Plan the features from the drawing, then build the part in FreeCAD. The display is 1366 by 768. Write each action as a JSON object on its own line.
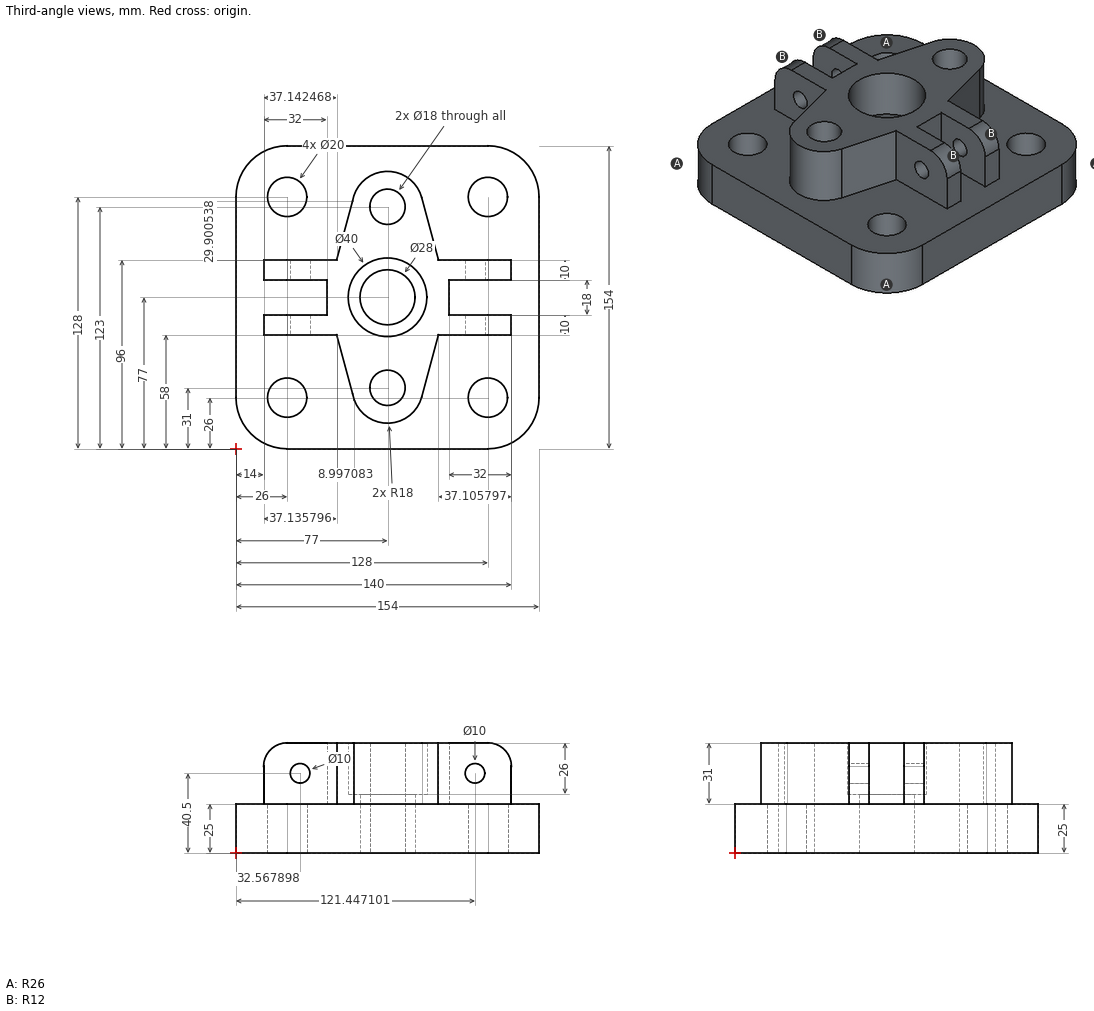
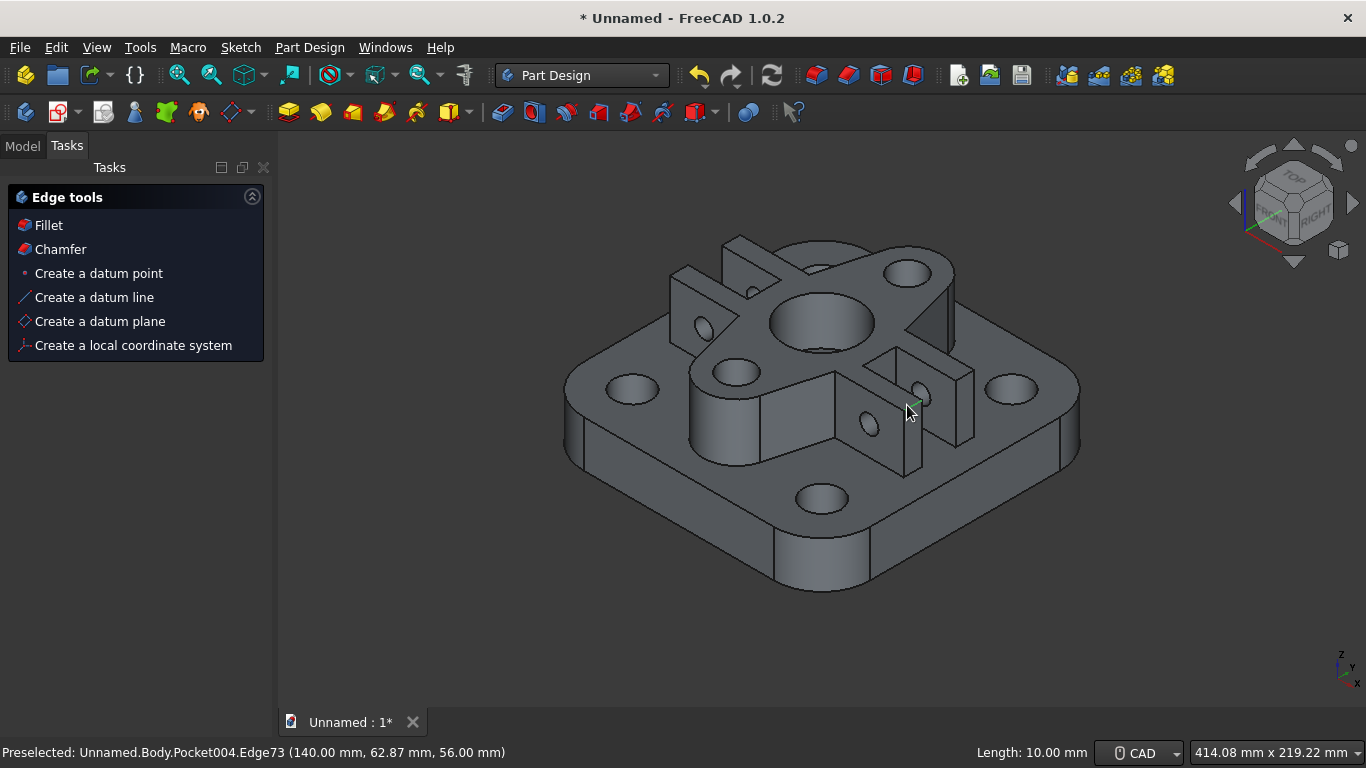
{"action": "left_click", "coordinate": [965, 374], "text": "ctrl"}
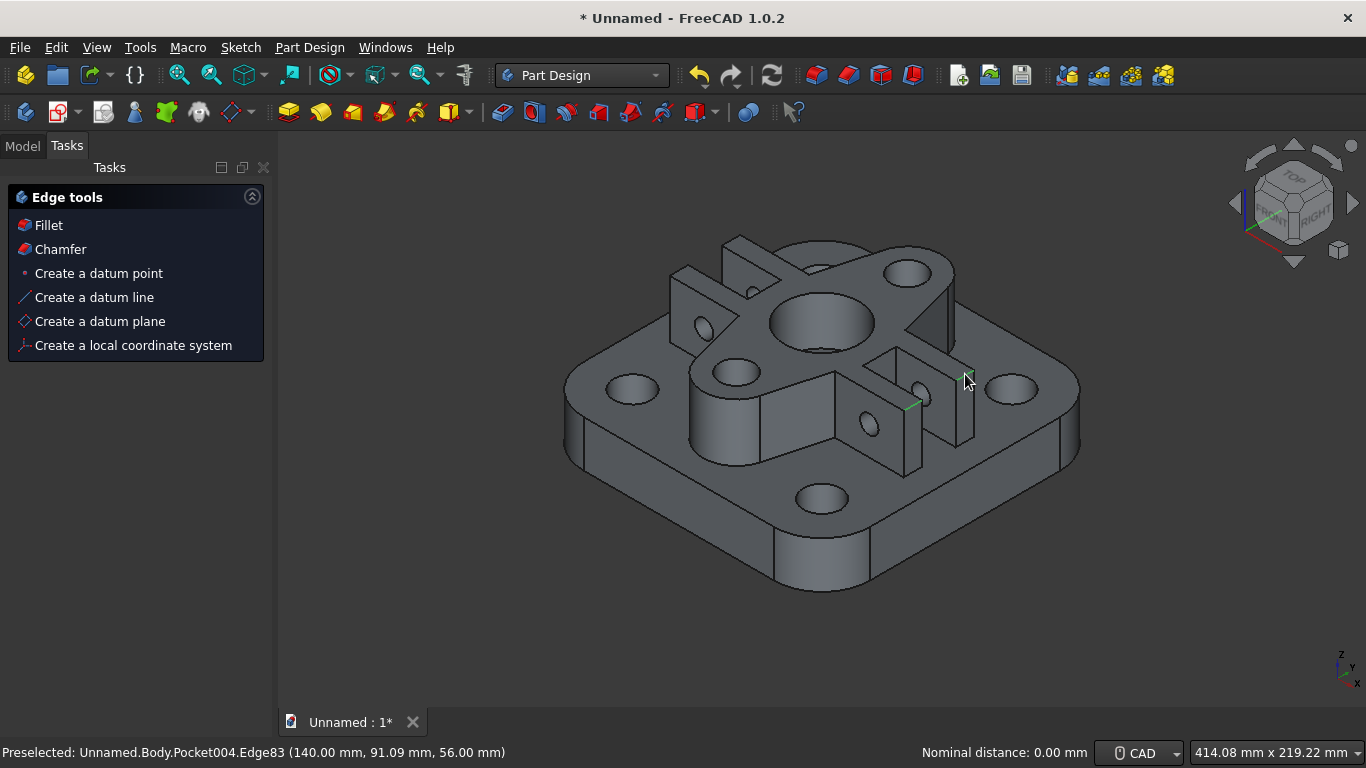
{"action": "key", "text": "2"}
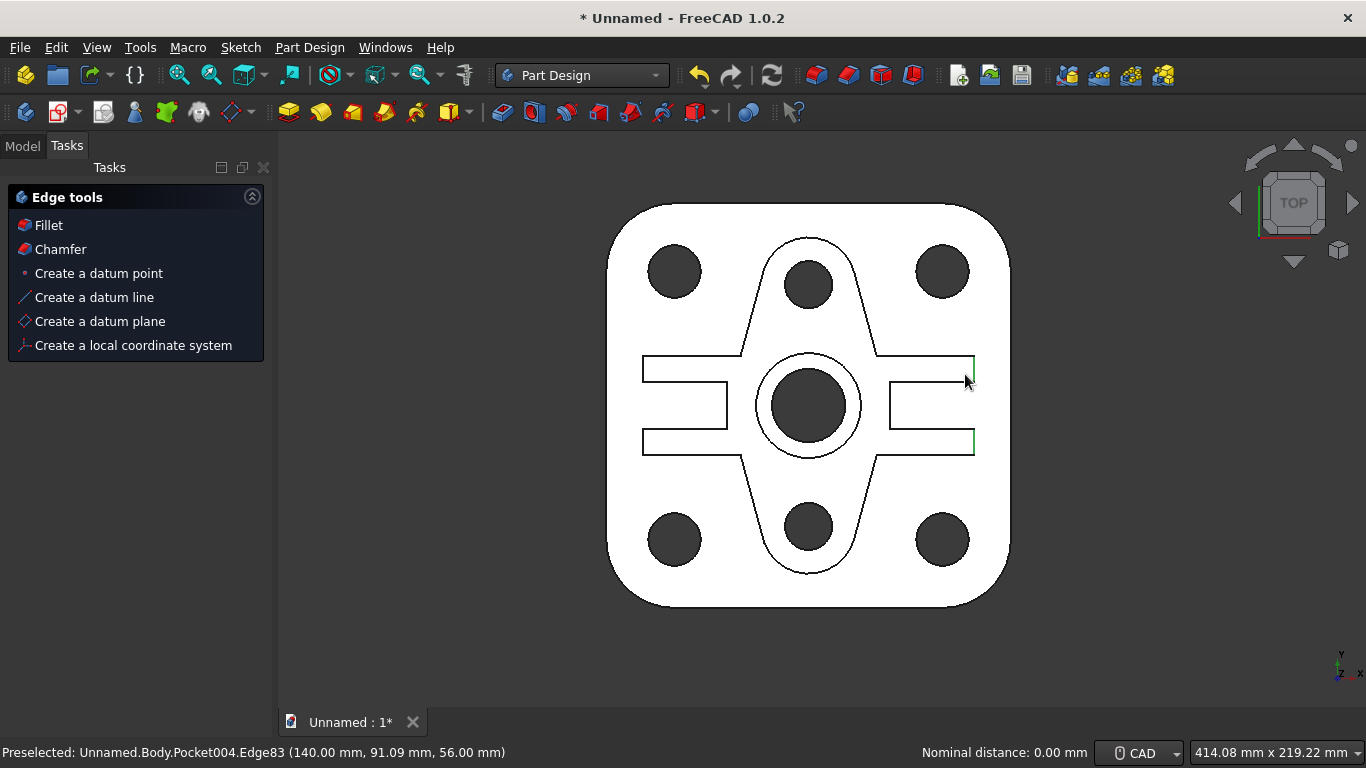
{"action": "left_click", "coordinate": [643, 368], "text": "ctrl"}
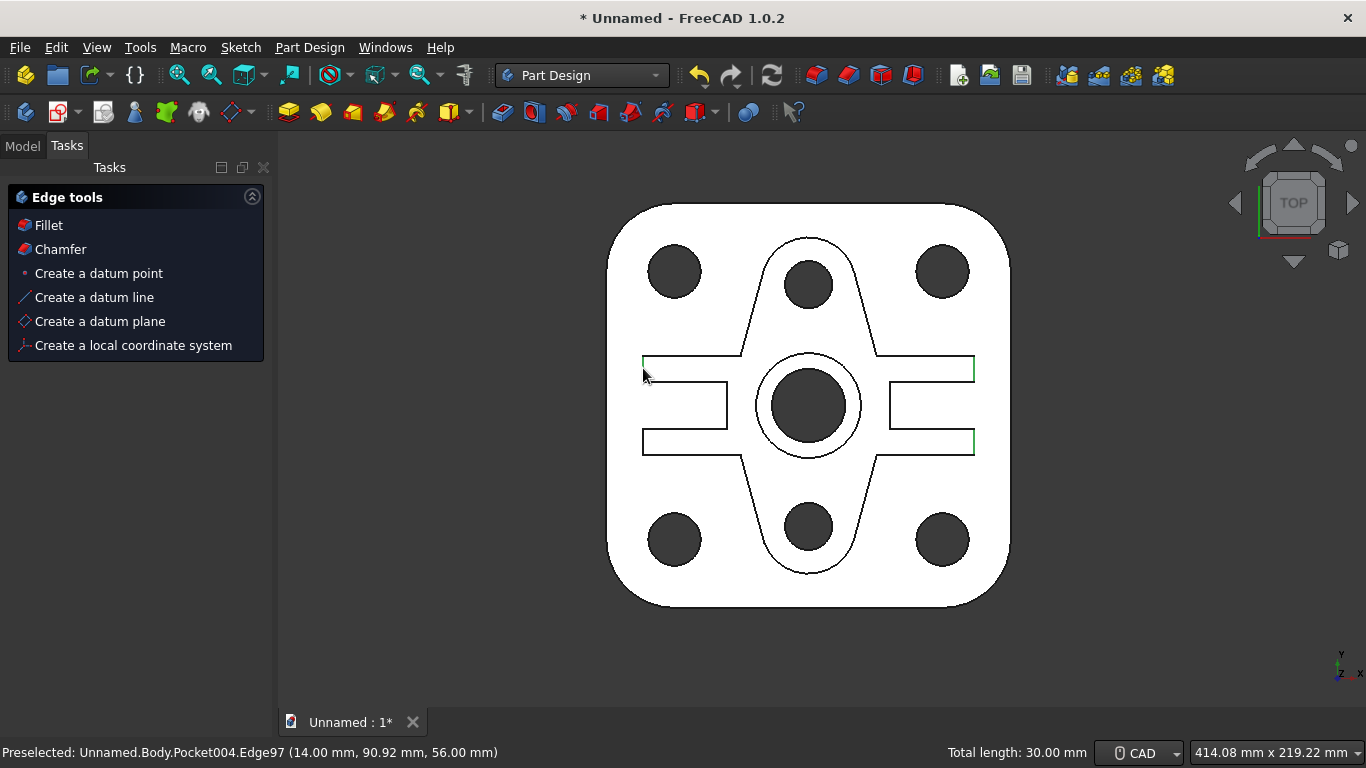
{"action": "left_click", "coordinate": [643, 441], "text": "ctrl"}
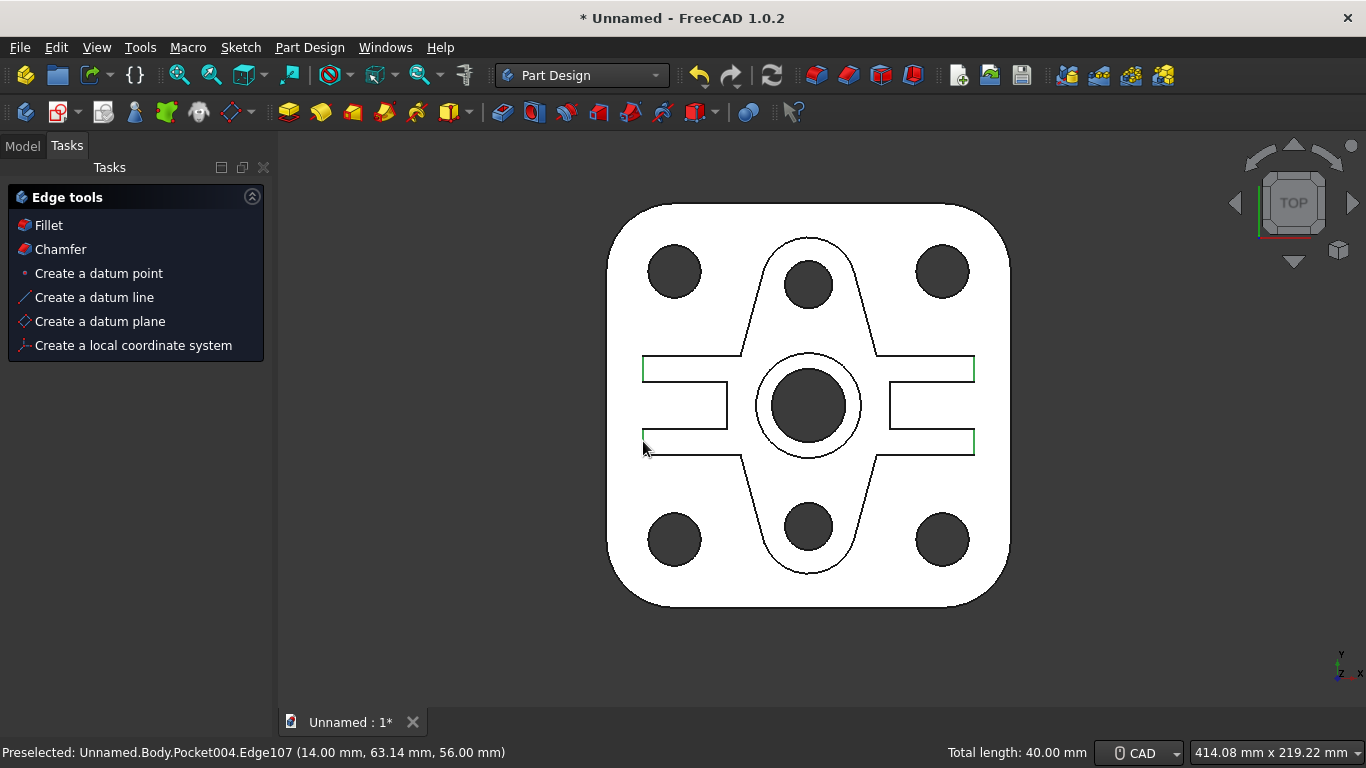
{"action": "left_click", "coordinate": [818, 76]}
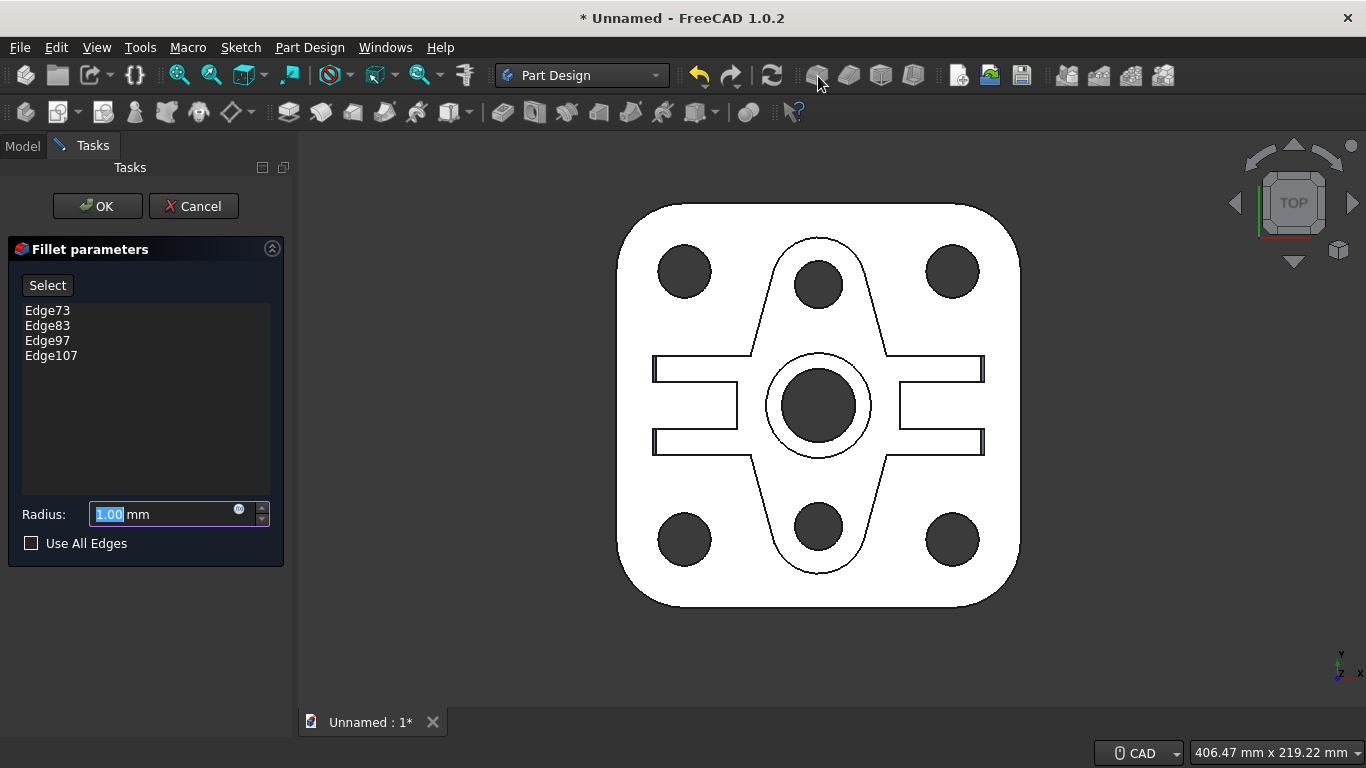
{"action": "type", "text": "12"}
{"action": "key", "text": "Tab"}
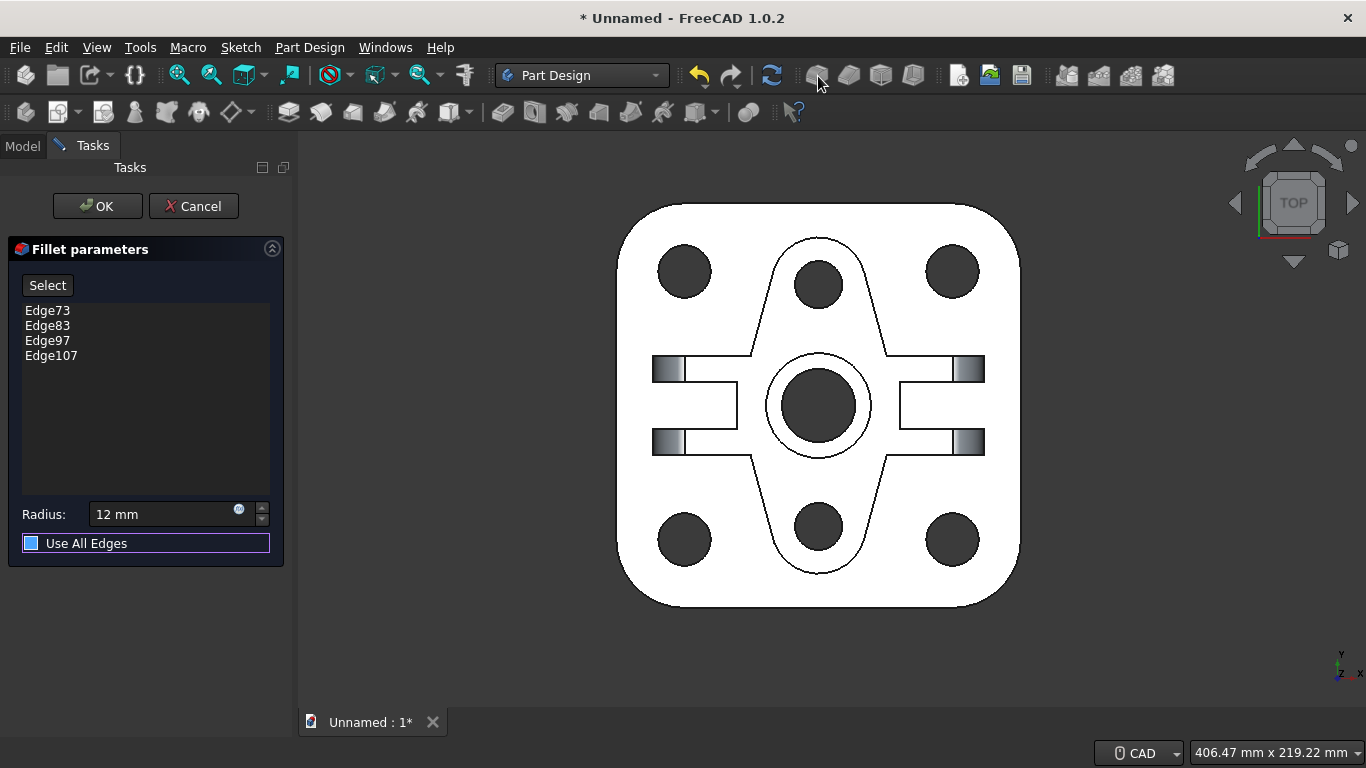
{"action": "left_click", "coordinate": [98, 206]}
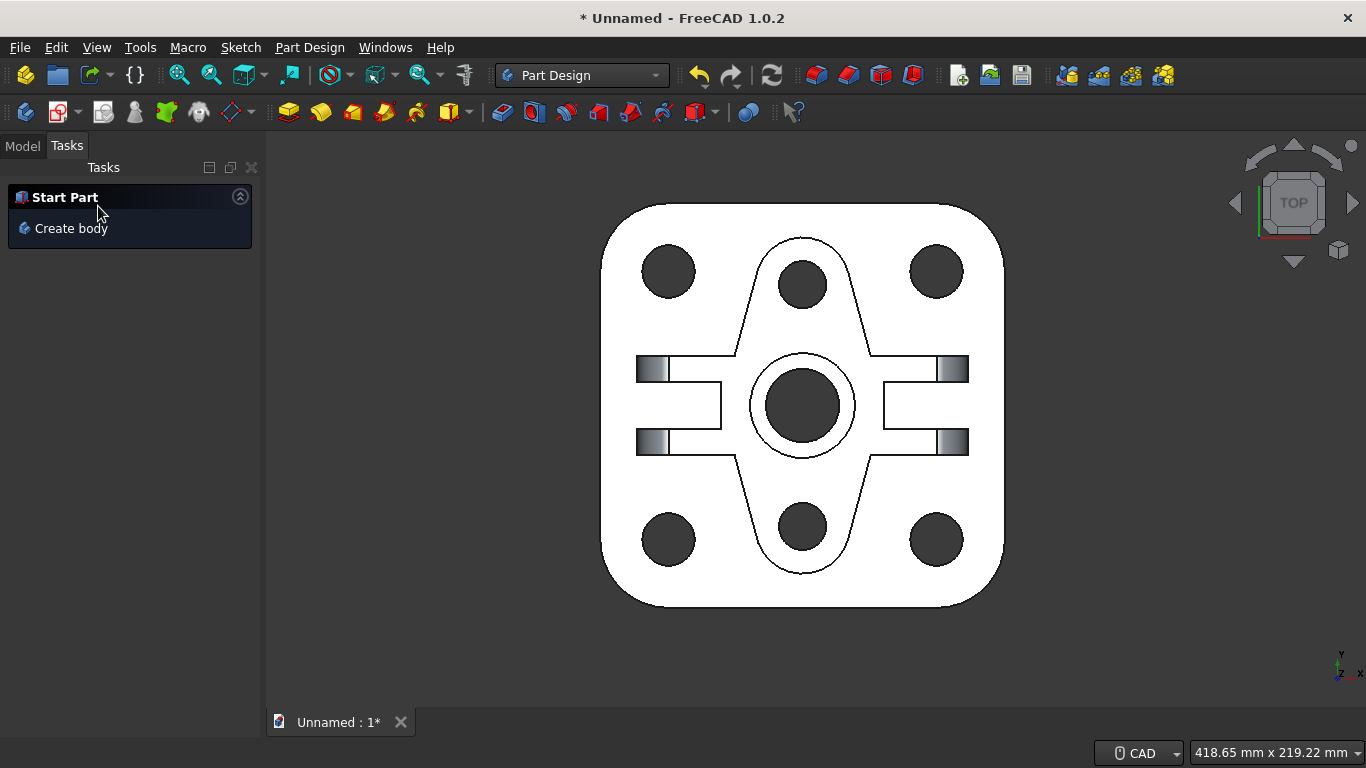
{"action": "key", "text": "0"}